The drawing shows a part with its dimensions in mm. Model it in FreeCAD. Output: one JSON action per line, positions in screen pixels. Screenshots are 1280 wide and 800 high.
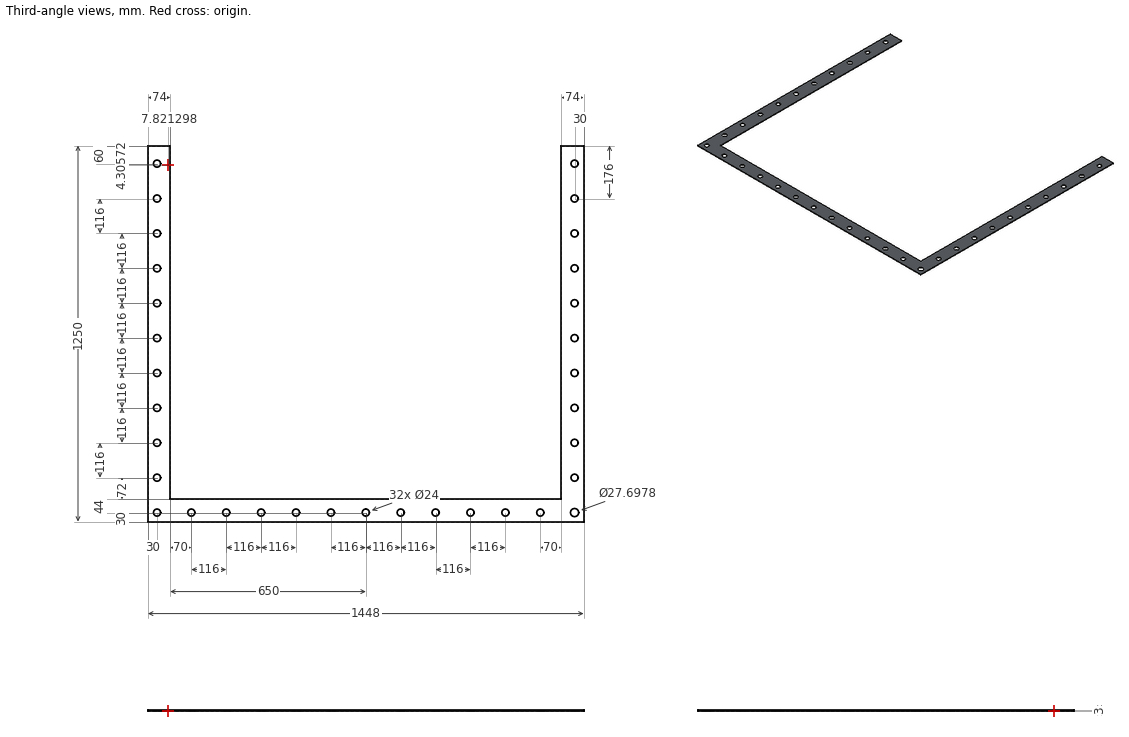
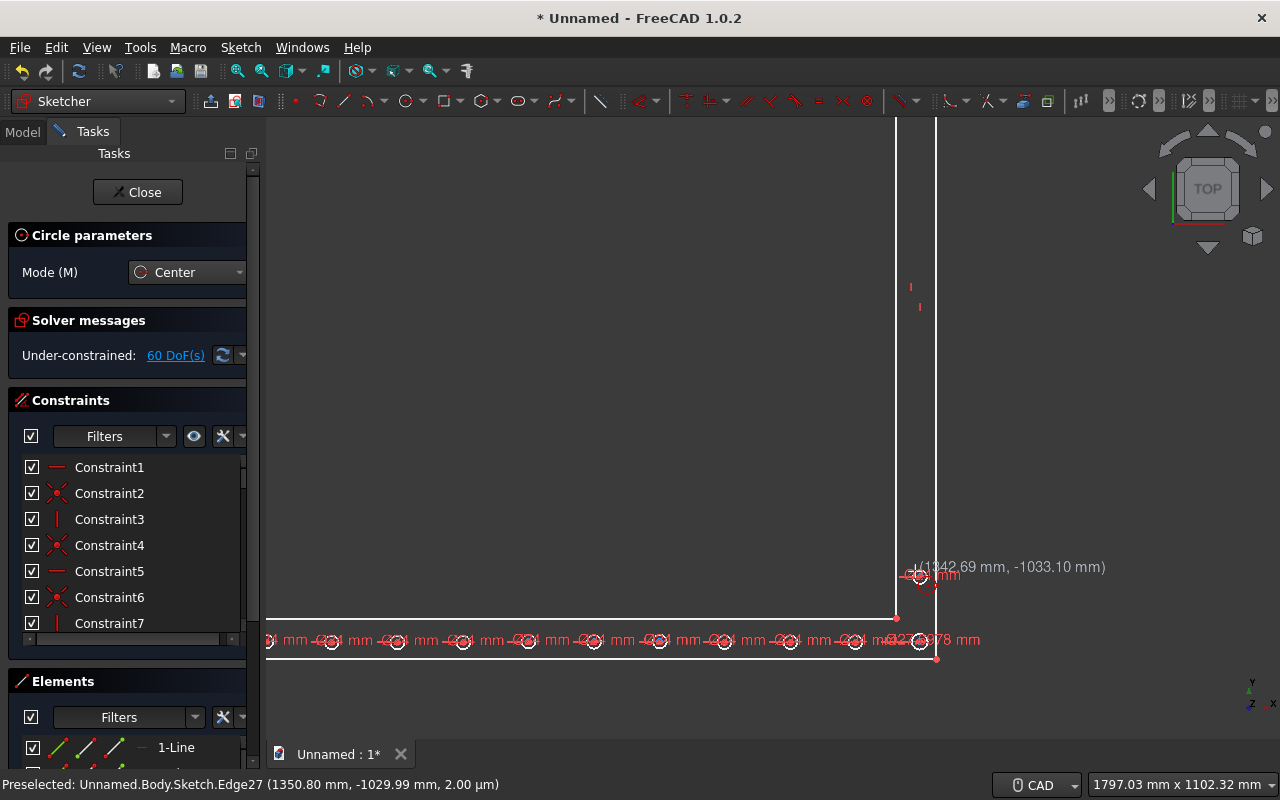
{"action": "scroll", "coordinate": [920, 510], "scroll_direction": "up", "scroll_amount": 7}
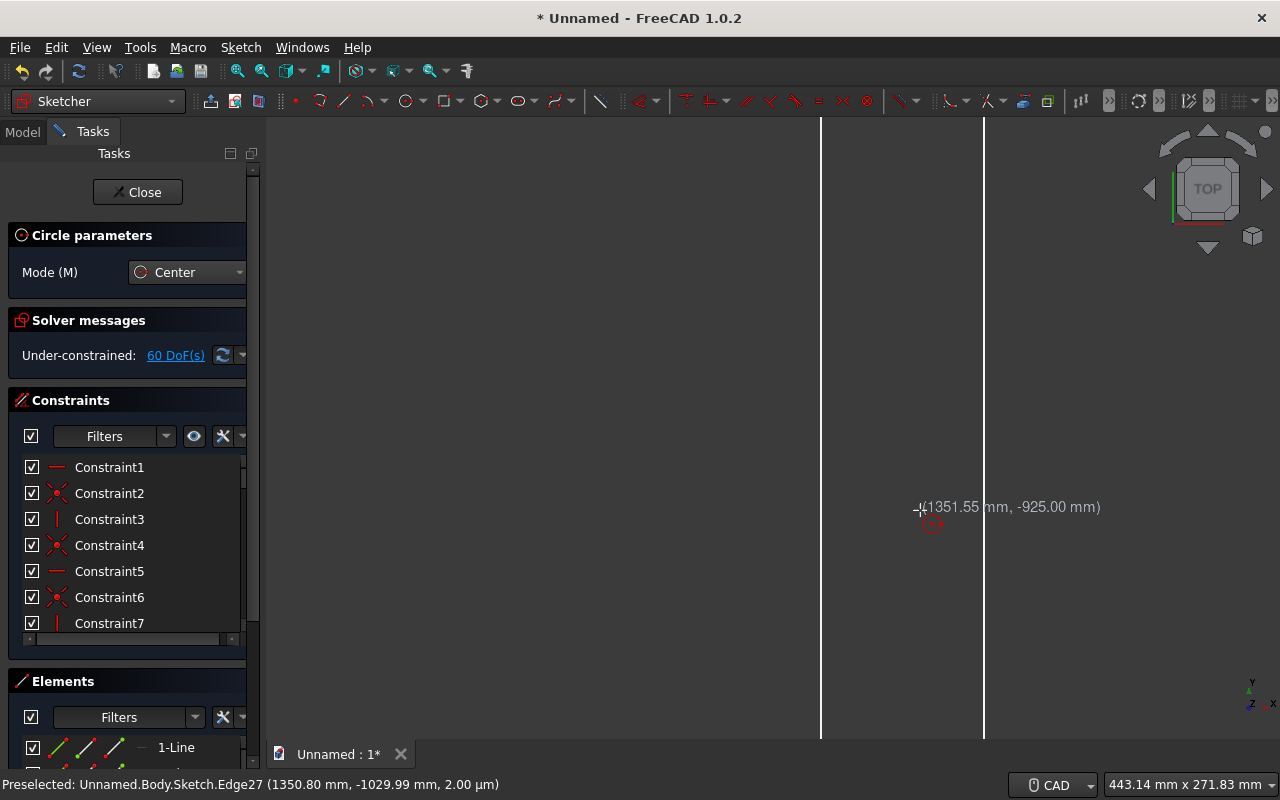
{"action": "scroll", "coordinate": [920, 545], "scroll_direction": "down", "scroll_amount": 10}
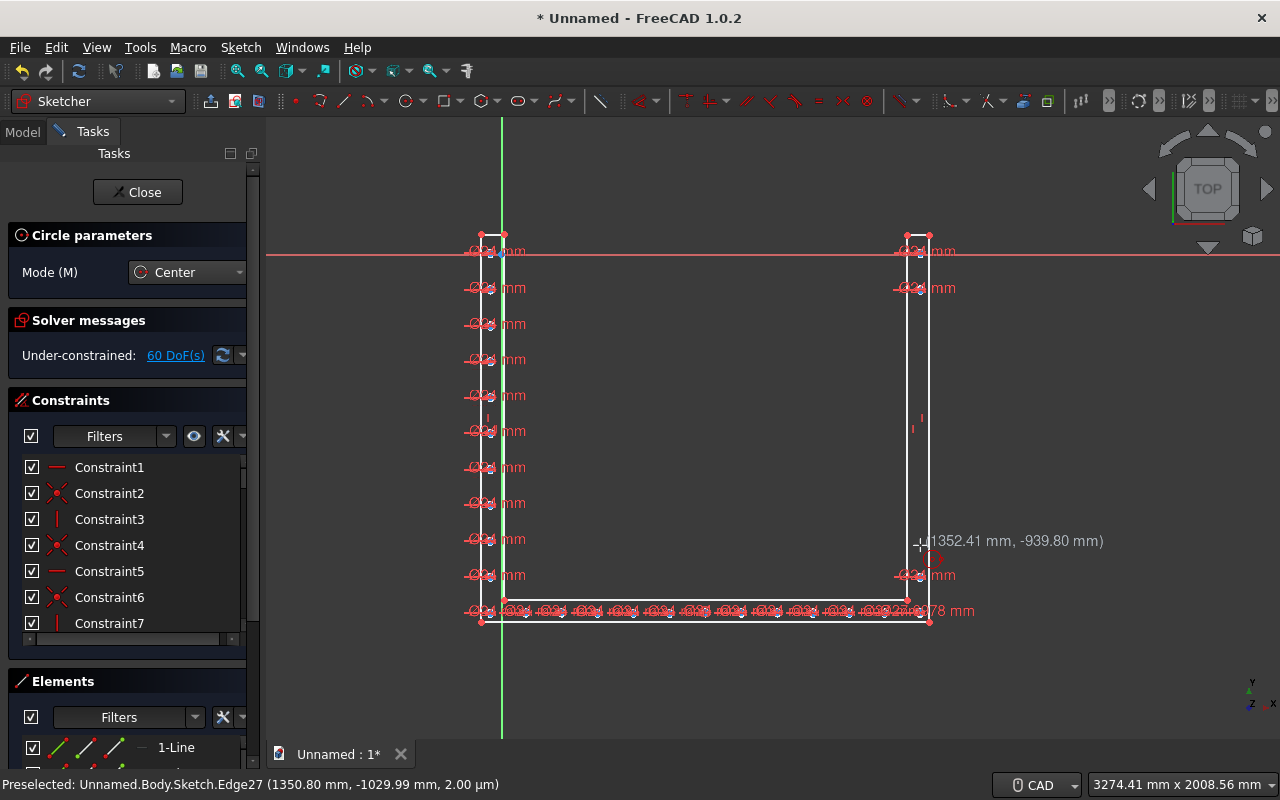
{"action": "scroll", "coordinate": [920, 541], "scroll_direction": "up", "scroll_amount": 3}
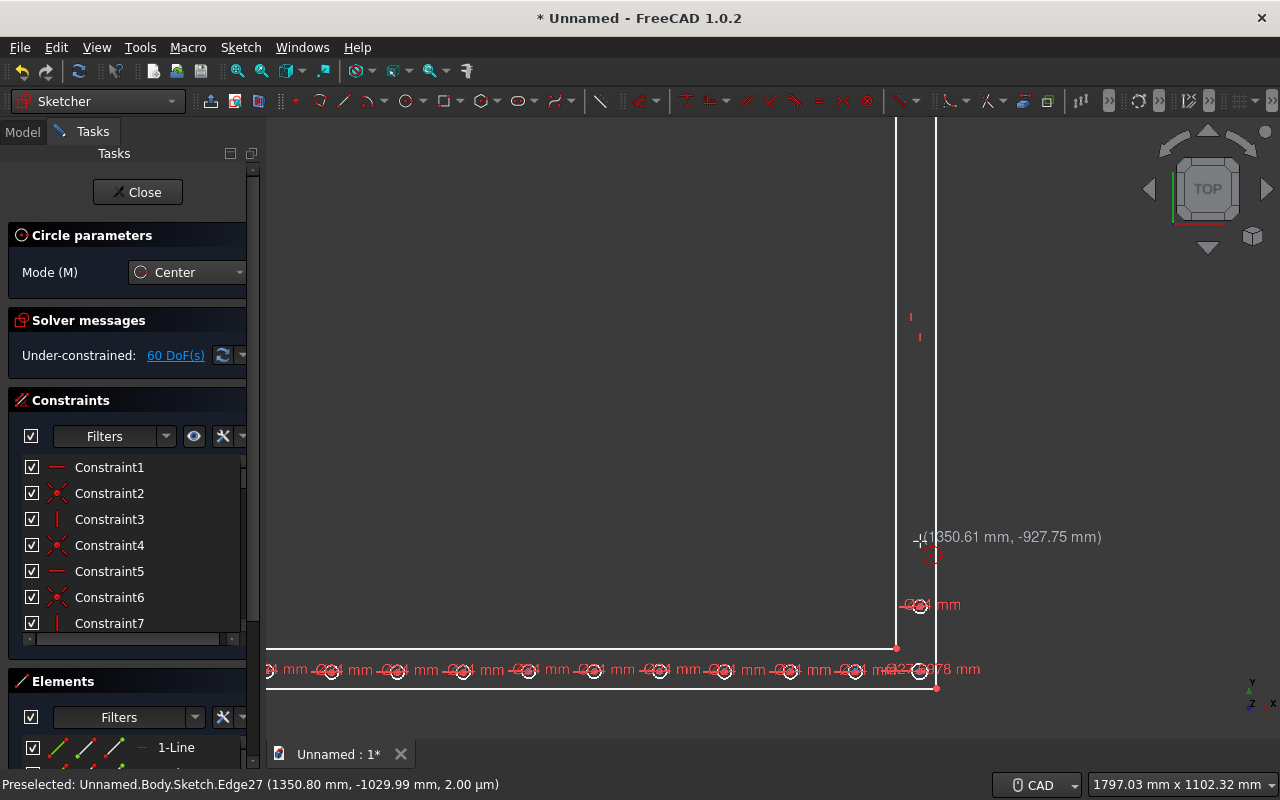
{"action": "left_click", "coordinate": [920, 540]}
{"action": "mouse_move", "coordinate": [915, 535]}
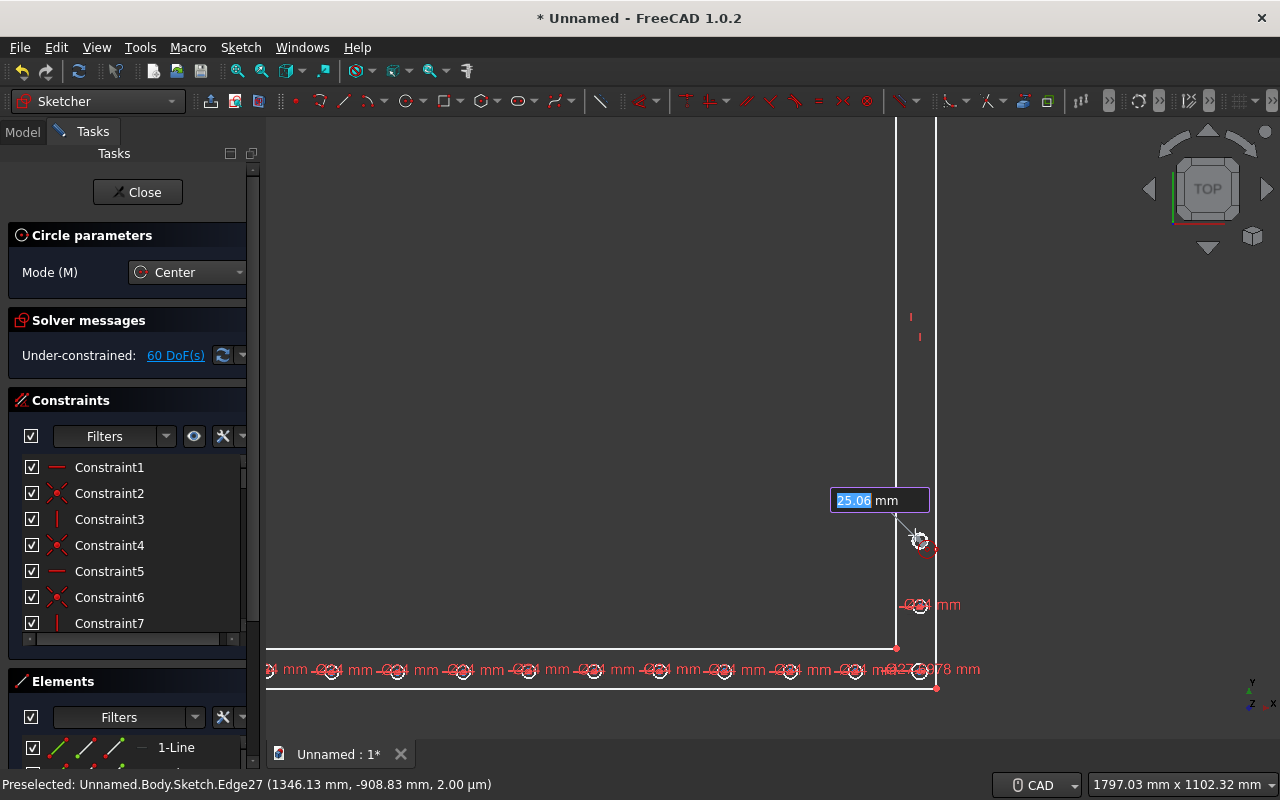
{"action": "type", "text": "24"}
{"action": "key", "text": "Return"}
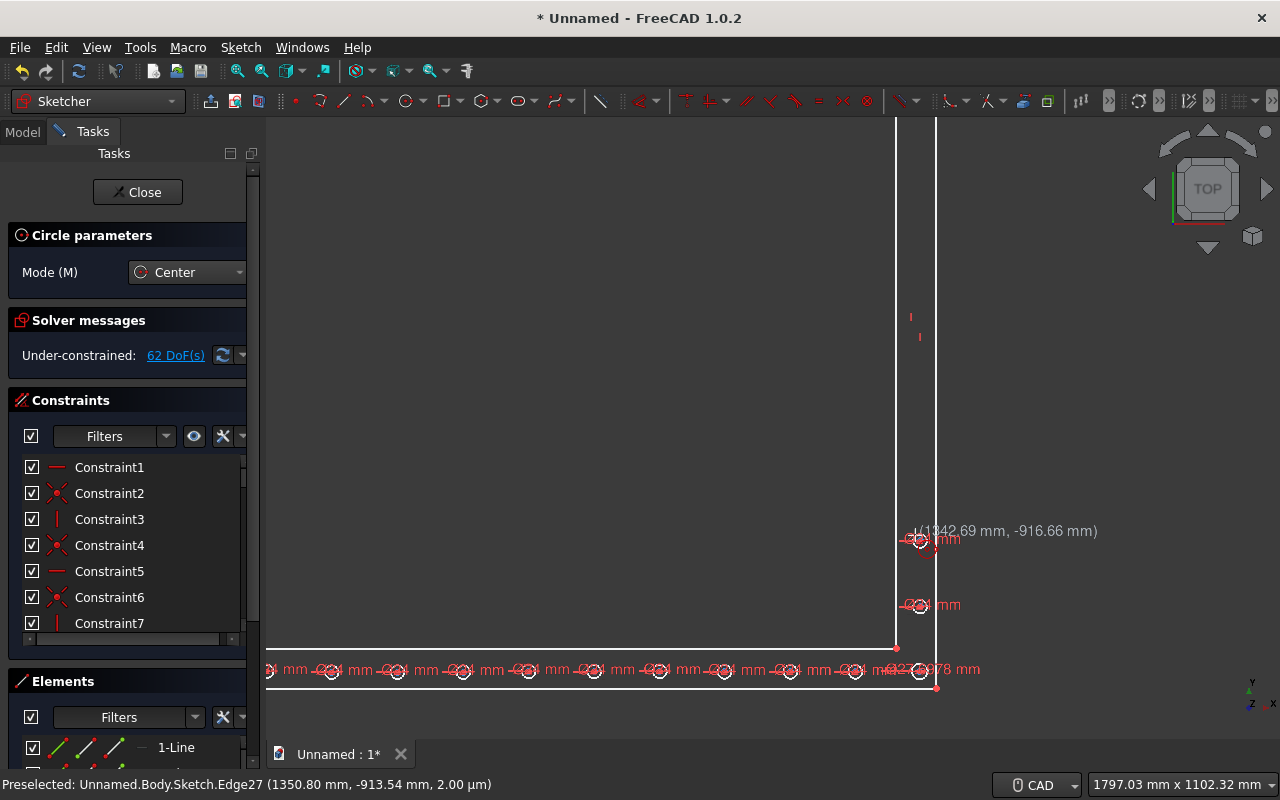
{"action": "scroll", "coordinate": [920, 475], "scroll_direction": "up", "scroll_amount": 7}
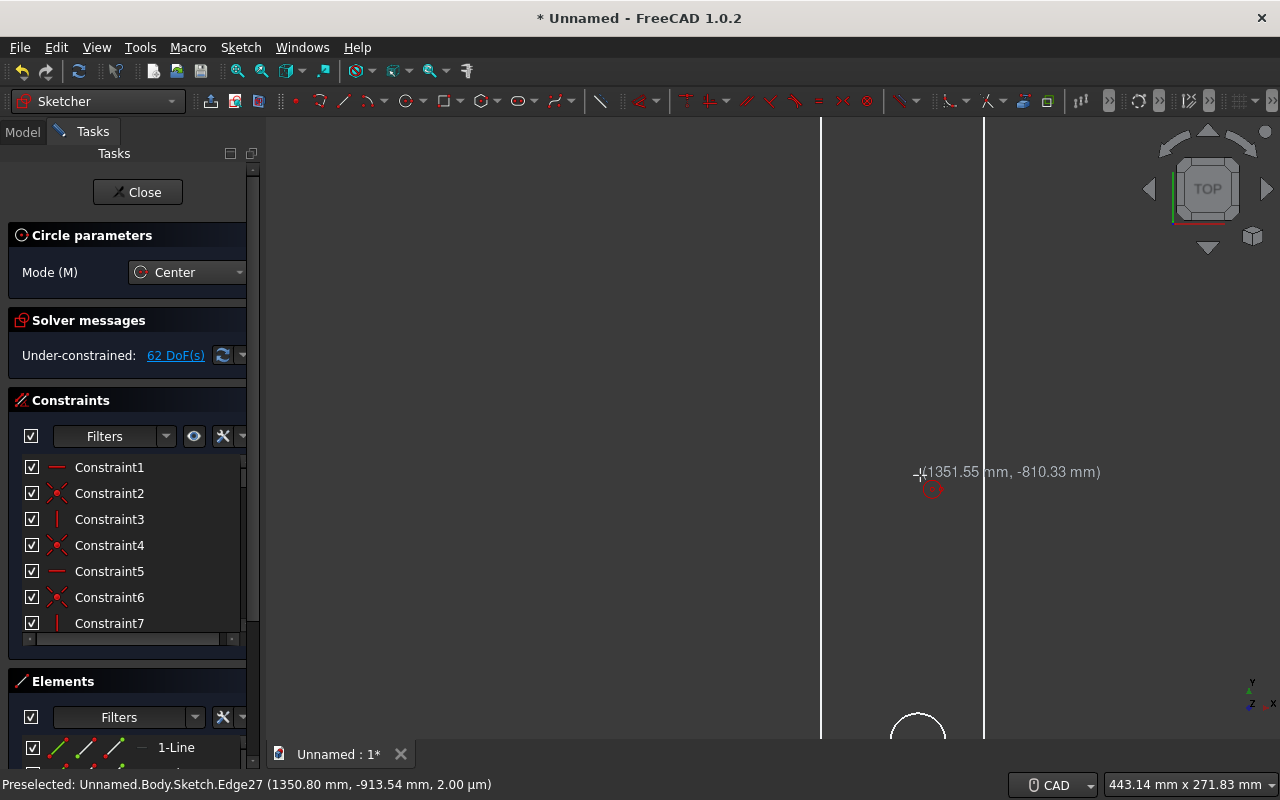
{"action": "scroll", "coordinate": [920, 510], "scroll_direction": "down", "scroll_amount": 10}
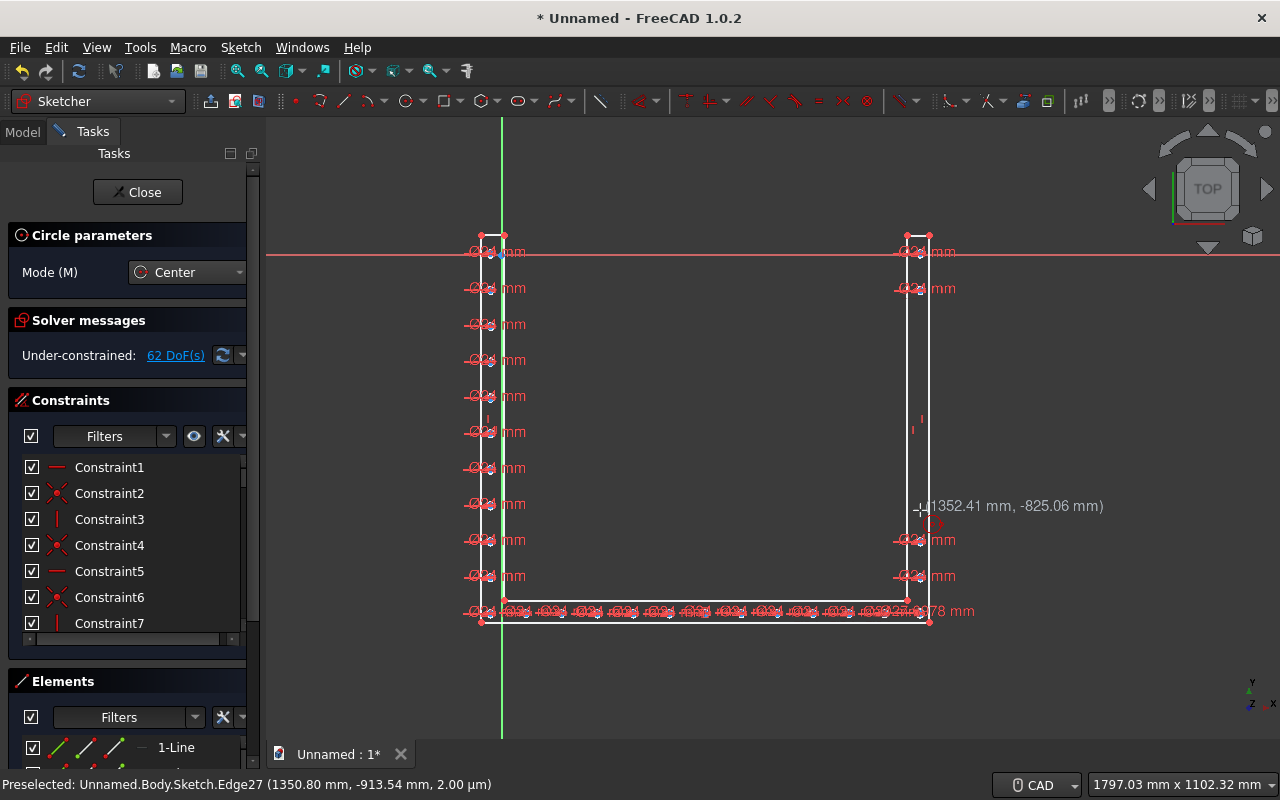
{"action": "scroll", "coordinate": [920, 505], "scroll_direction": "up", "scroll_amount": 3}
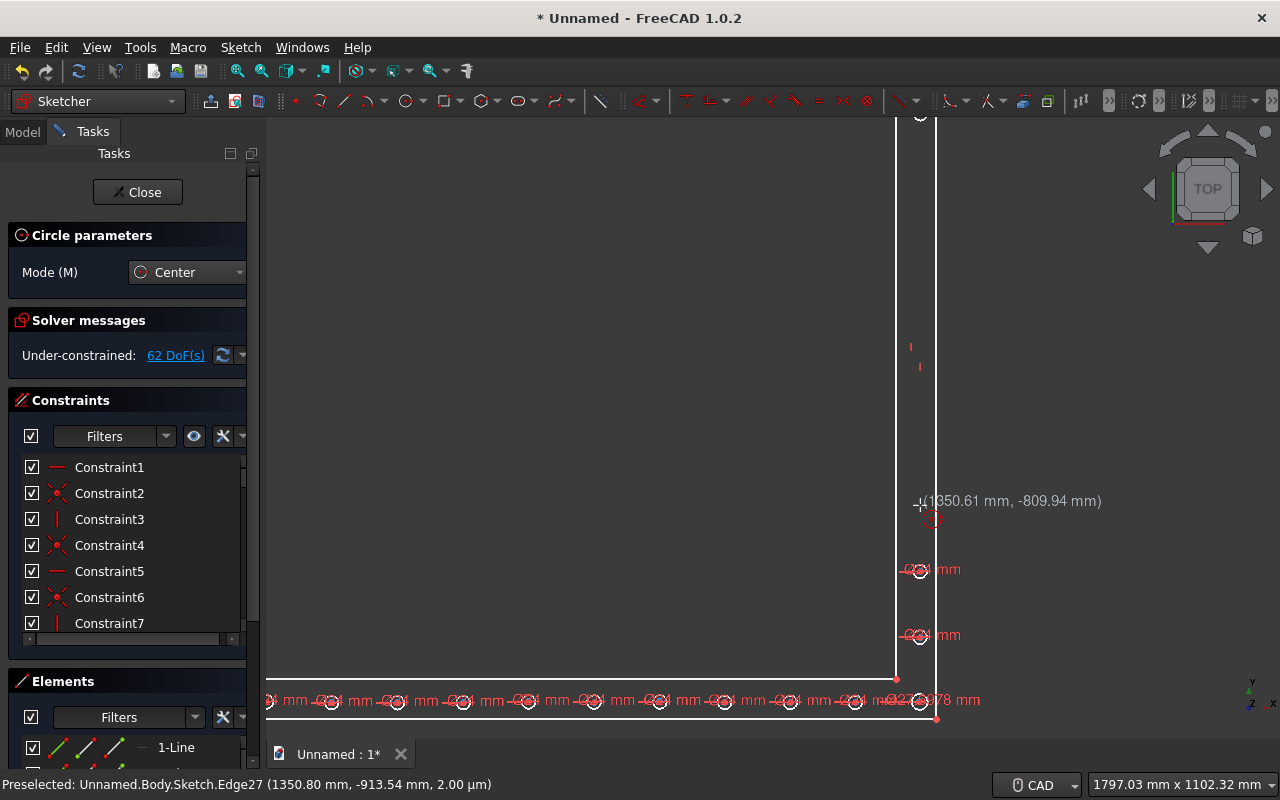
{"action": "left_click", "coordinate": [920, 505]}
{"action": "mouse_move", "coordinate": [915, 500]}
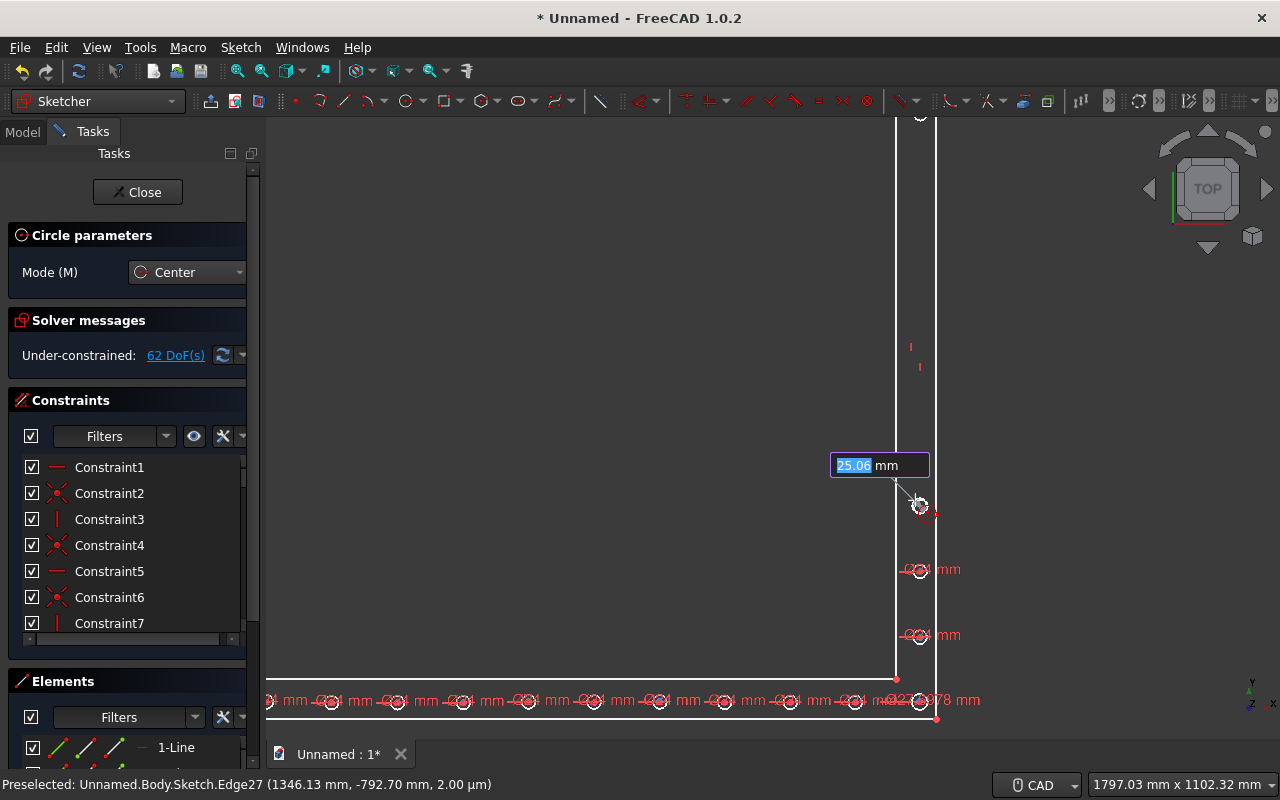
{"action": "type", "text": "24"}
{"action": "key", "text": "Return"}